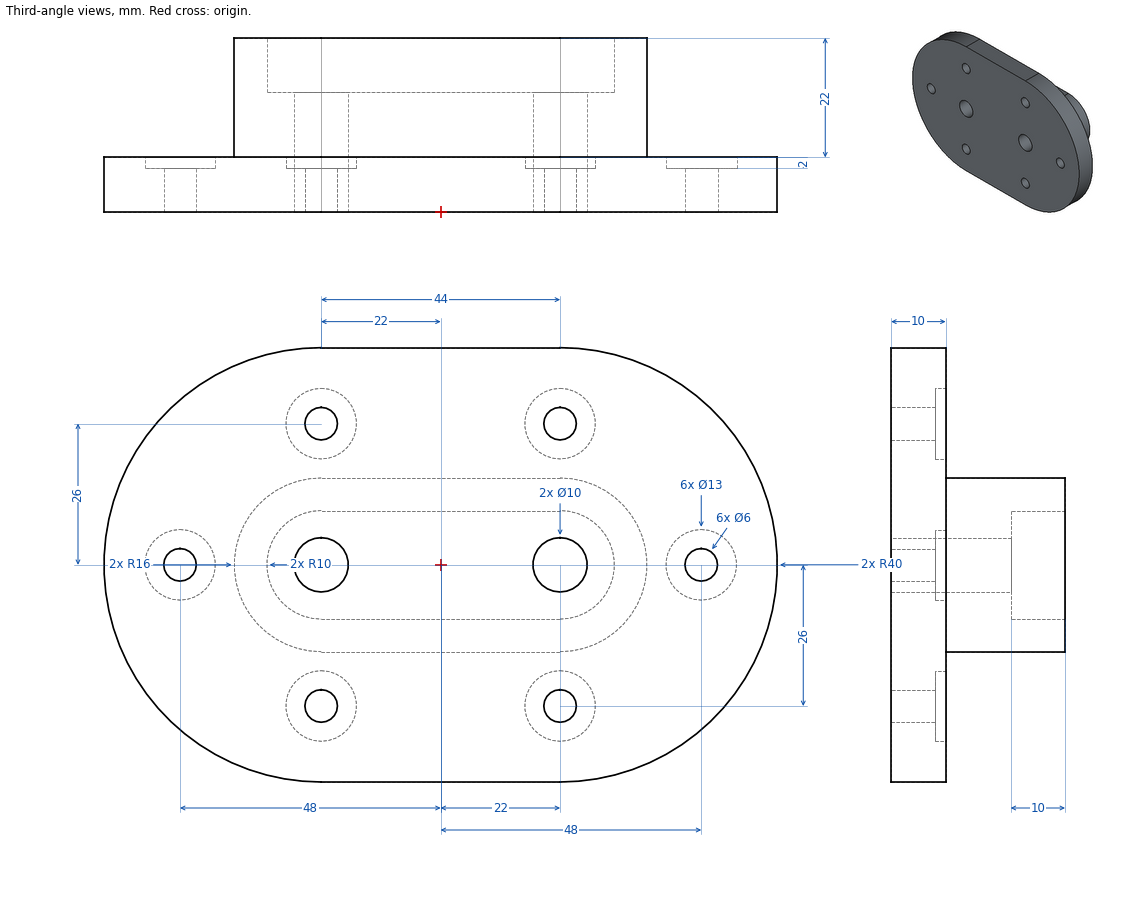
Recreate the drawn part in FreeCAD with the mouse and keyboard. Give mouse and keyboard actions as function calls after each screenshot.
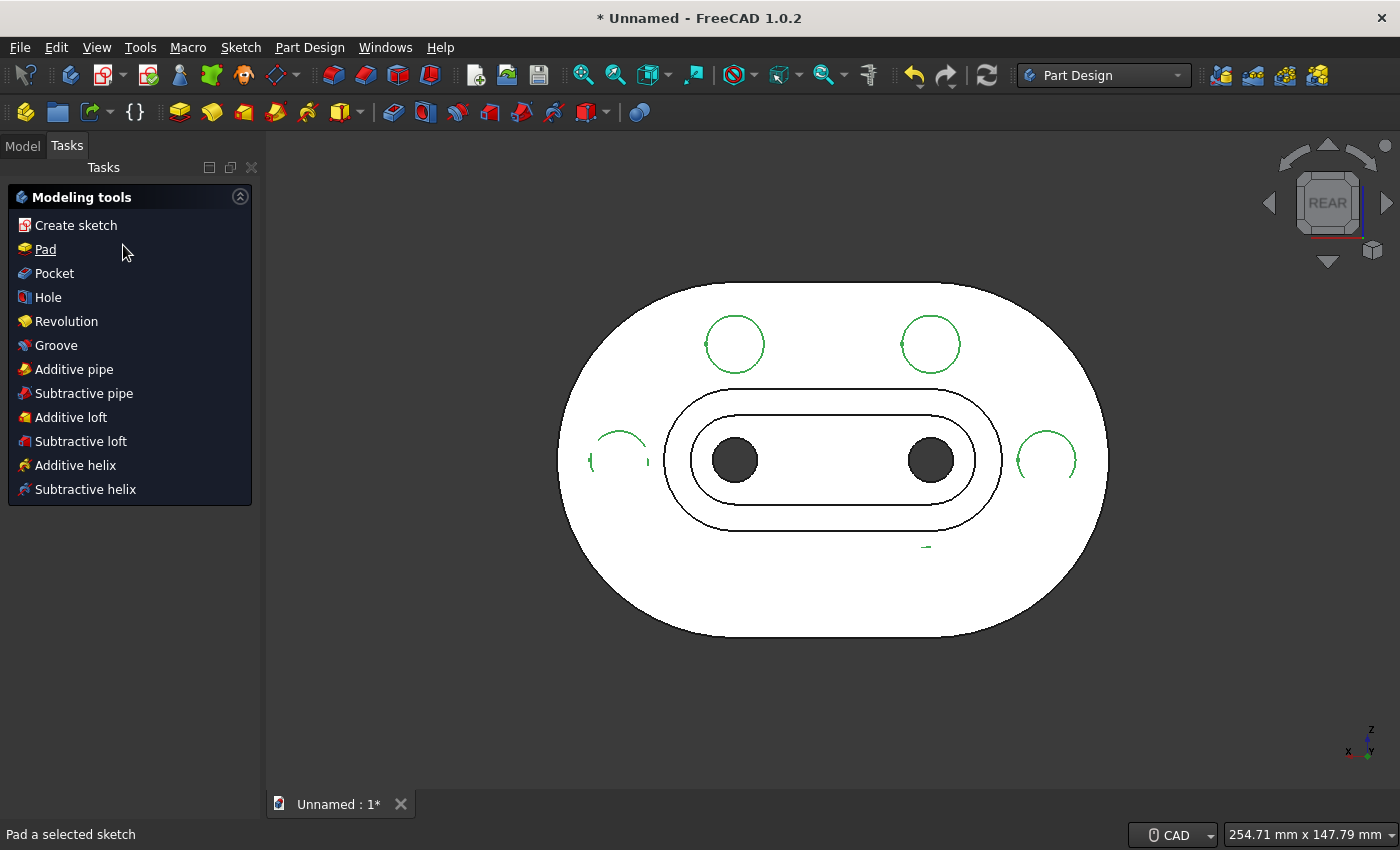
click(394, 112)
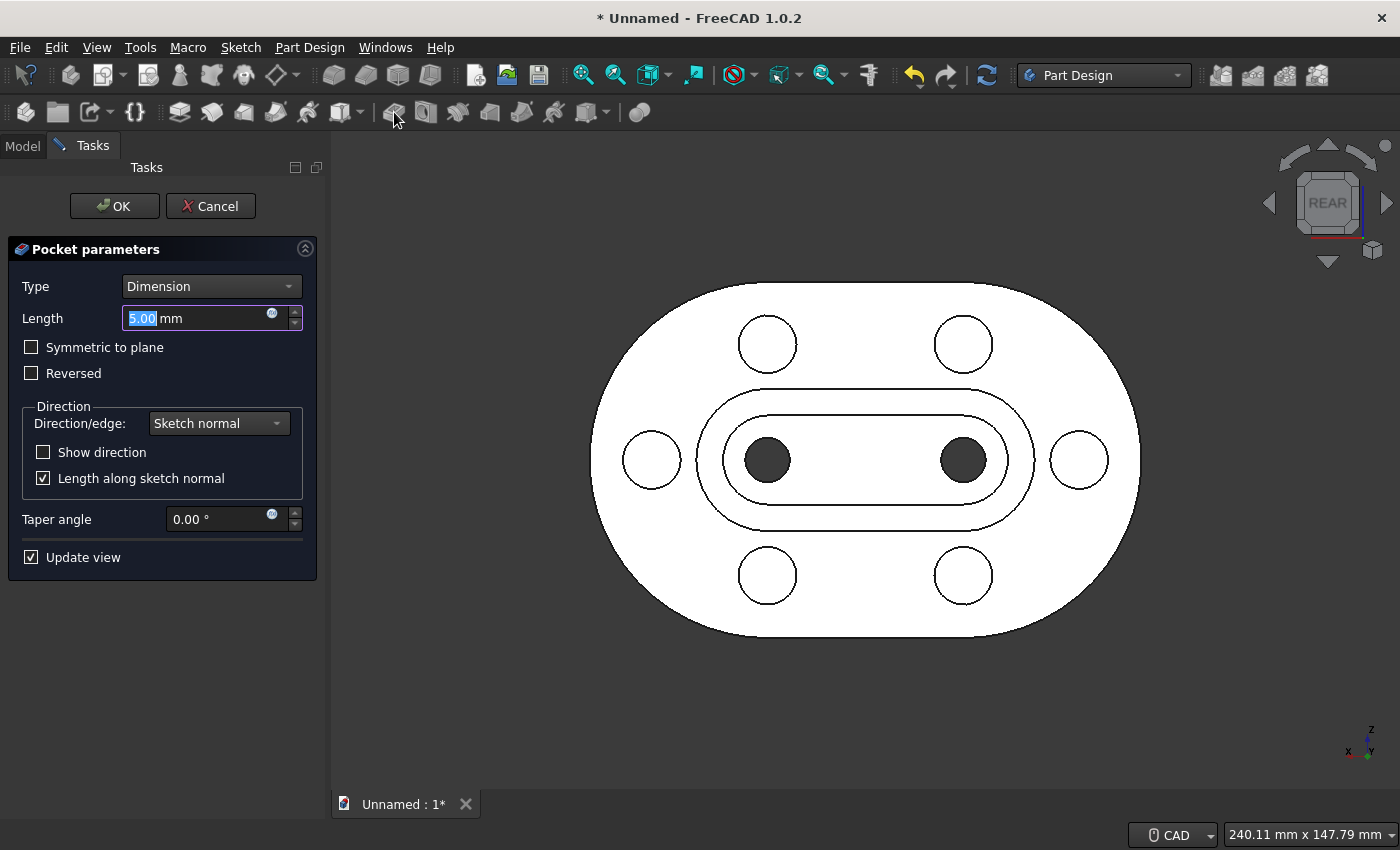
text(2)
key(Tab)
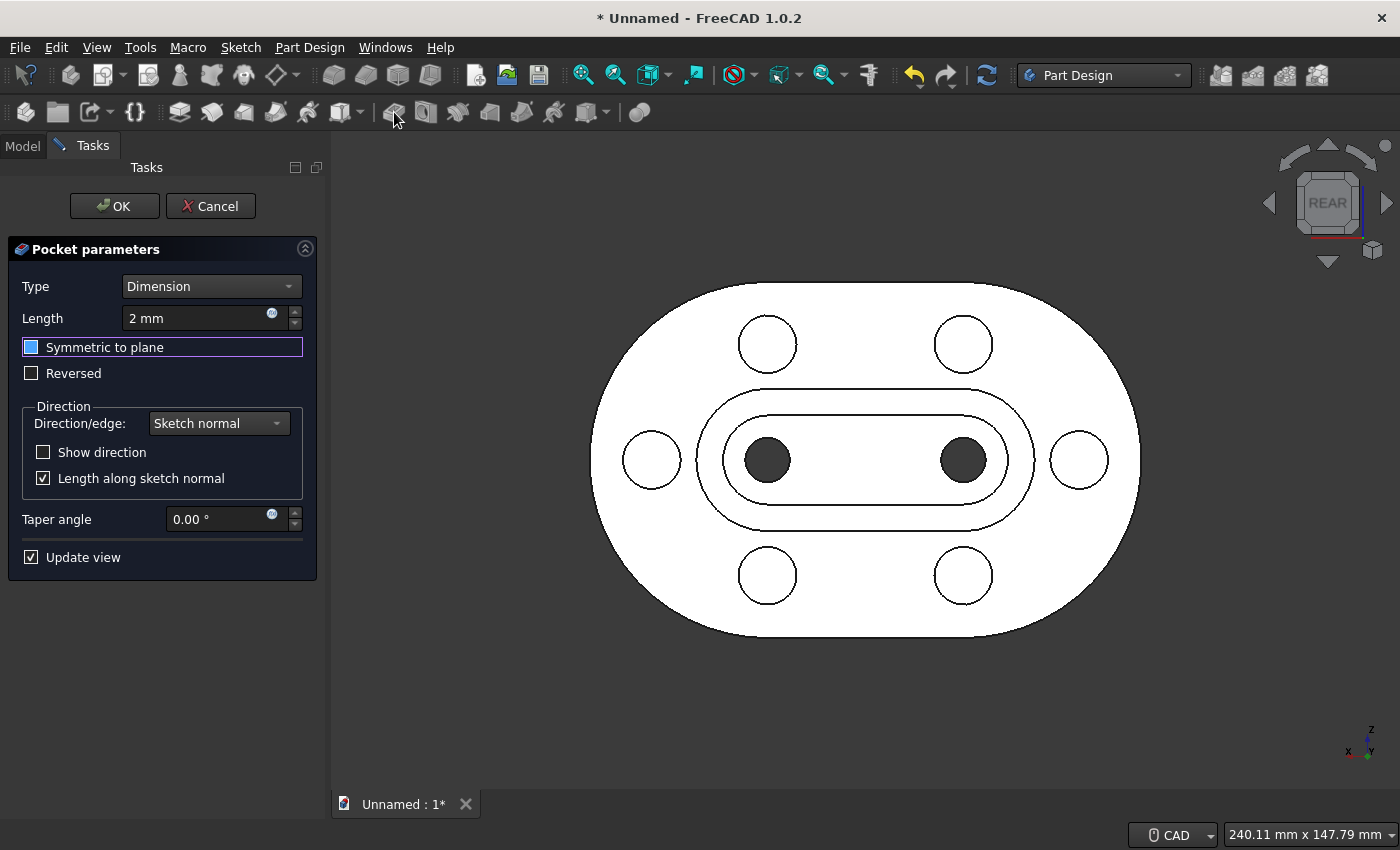
click(115, 206)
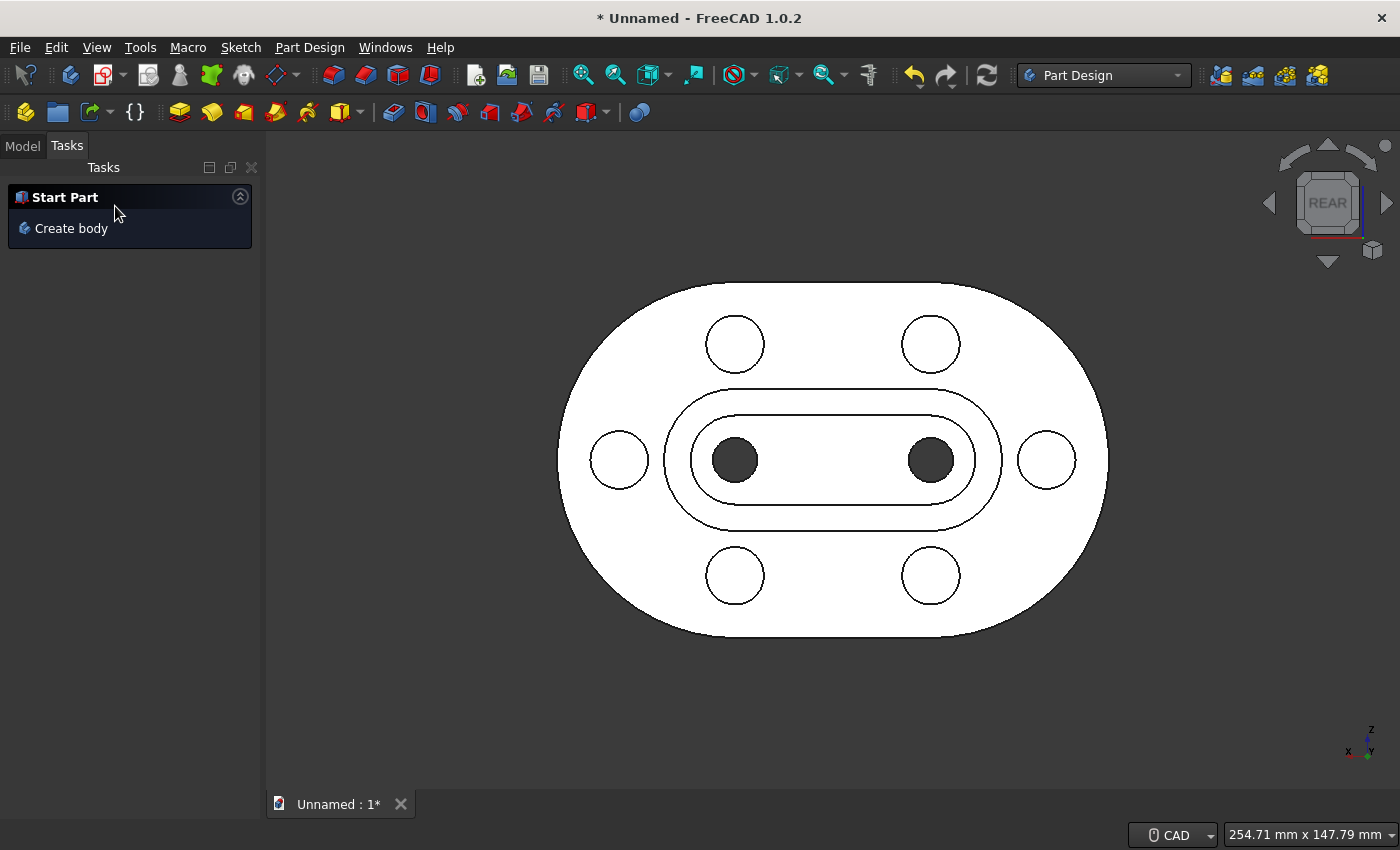
click(619, 459)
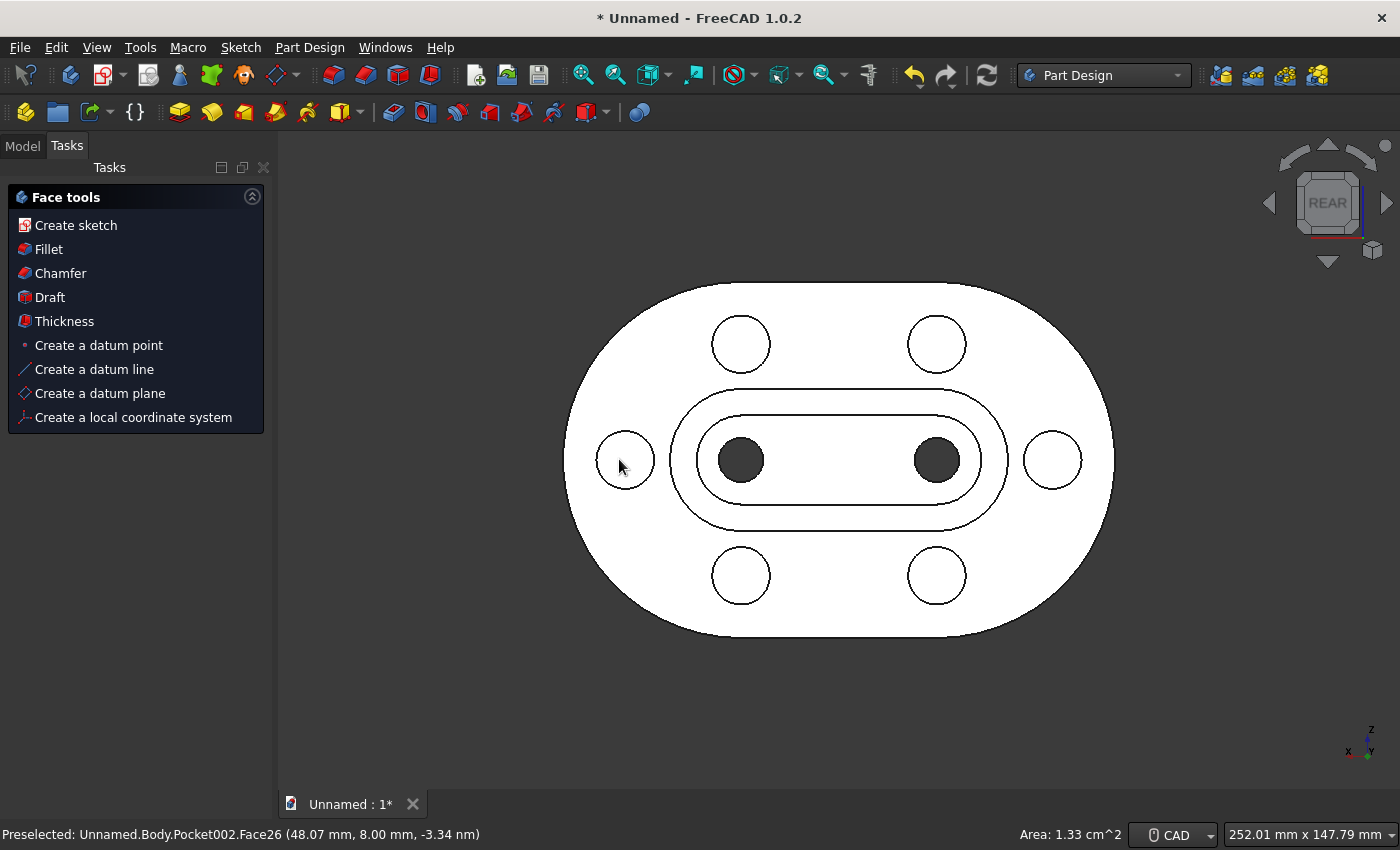
click(104, 76)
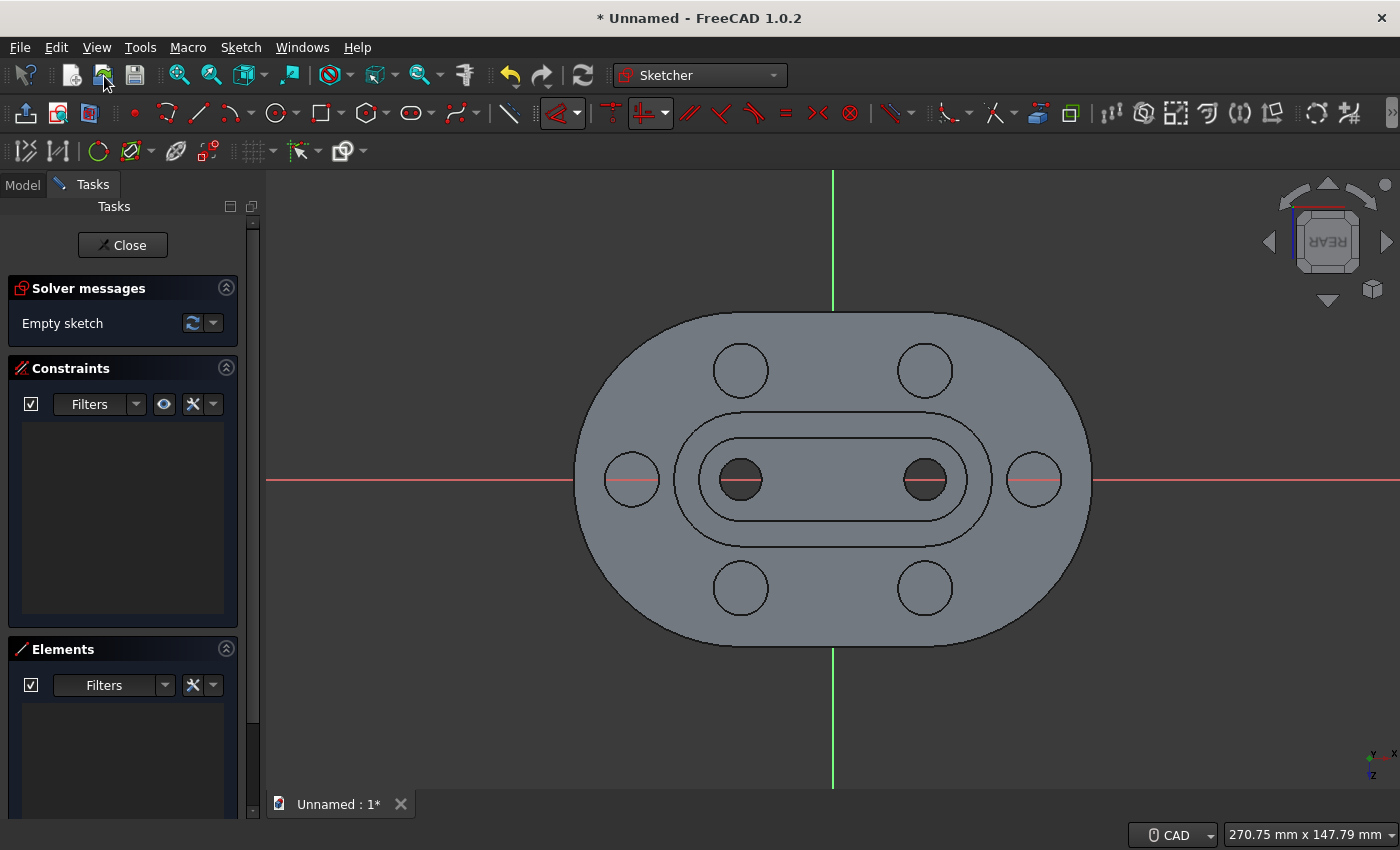
key(q)
key(s)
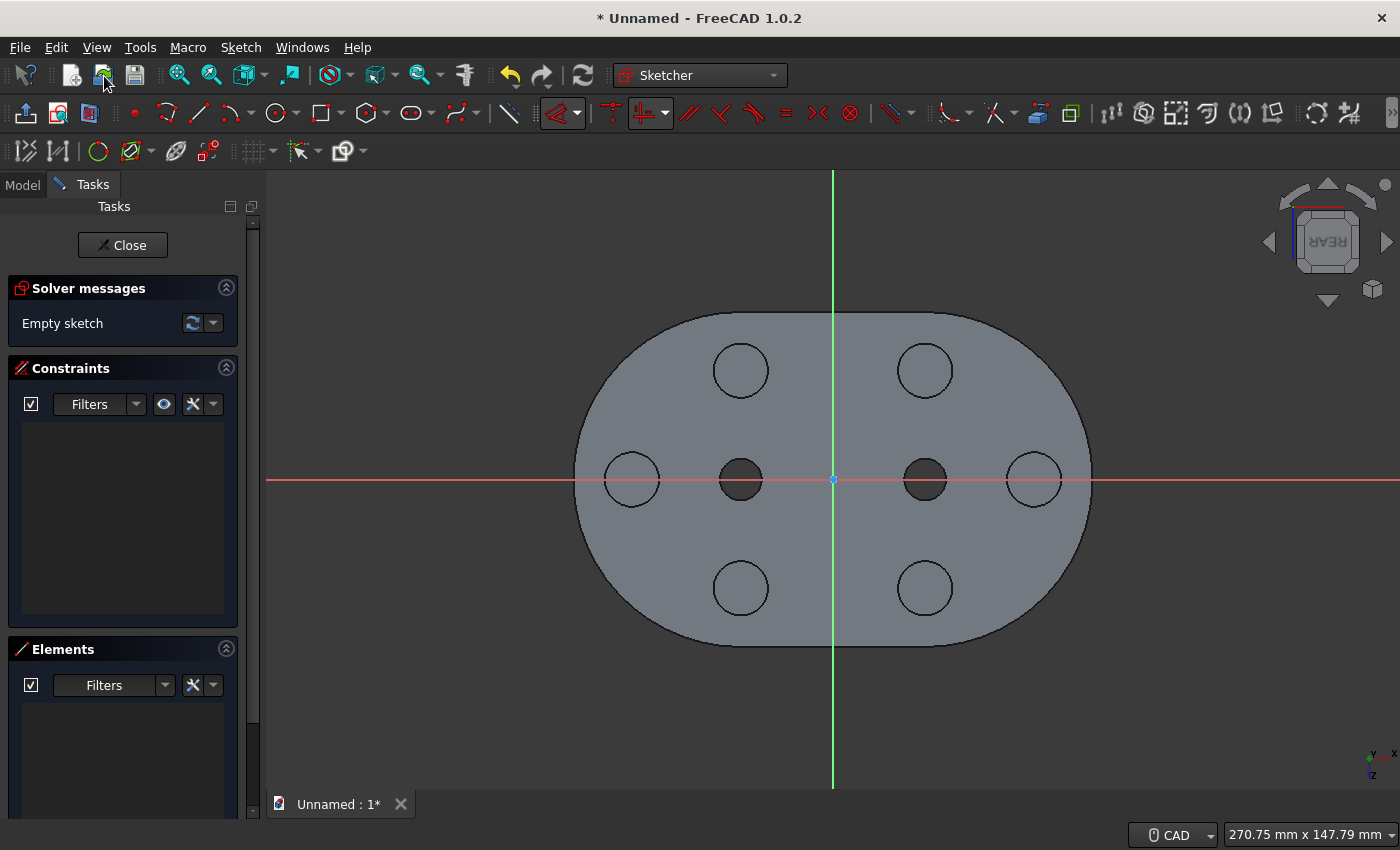
scroll(972, 479, up, 2)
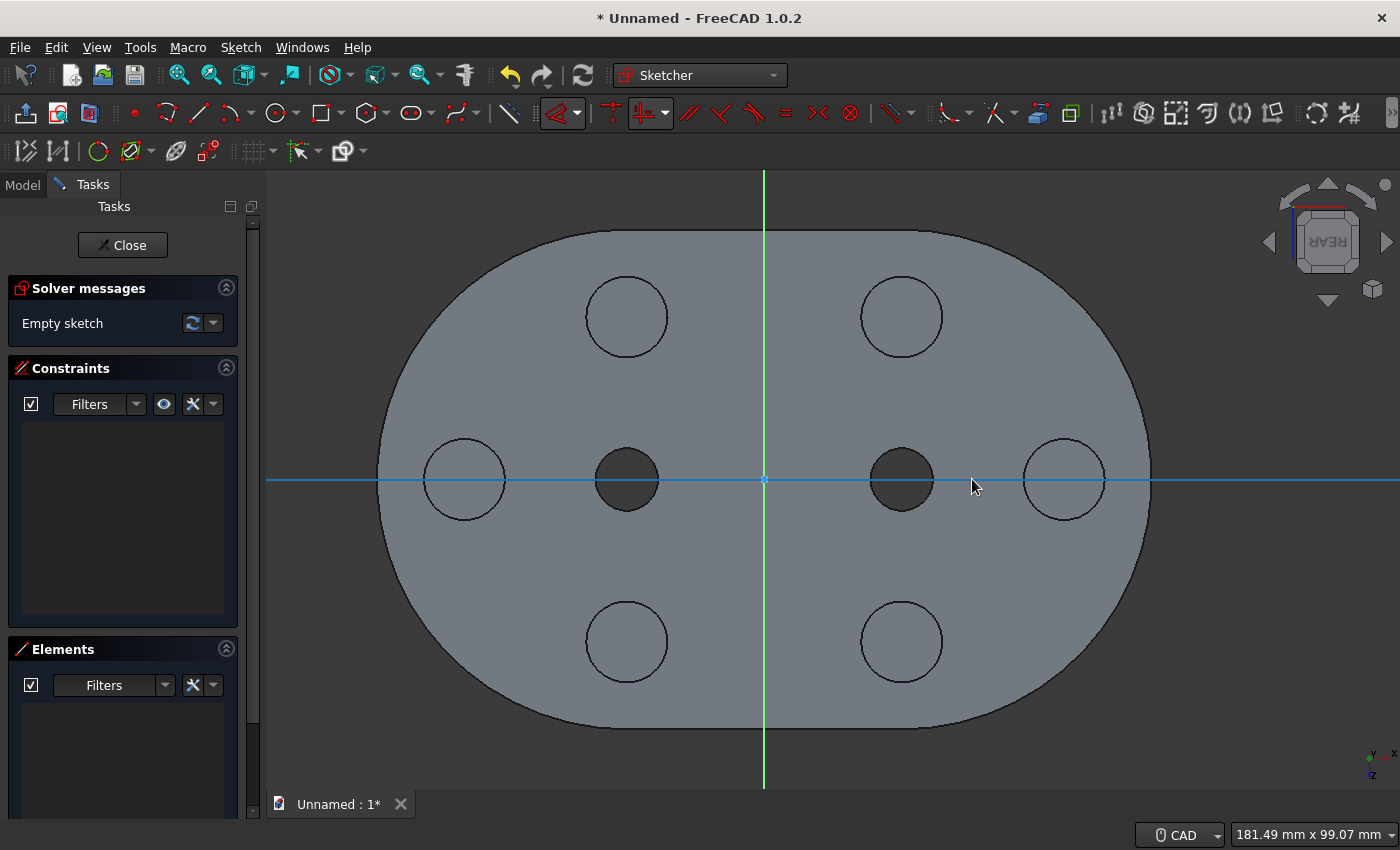
click(276, 114)